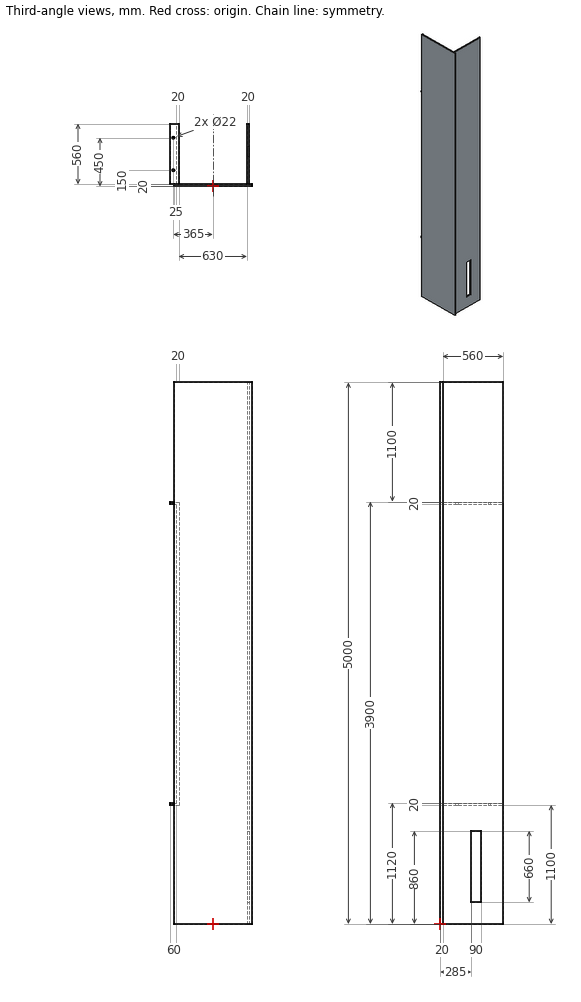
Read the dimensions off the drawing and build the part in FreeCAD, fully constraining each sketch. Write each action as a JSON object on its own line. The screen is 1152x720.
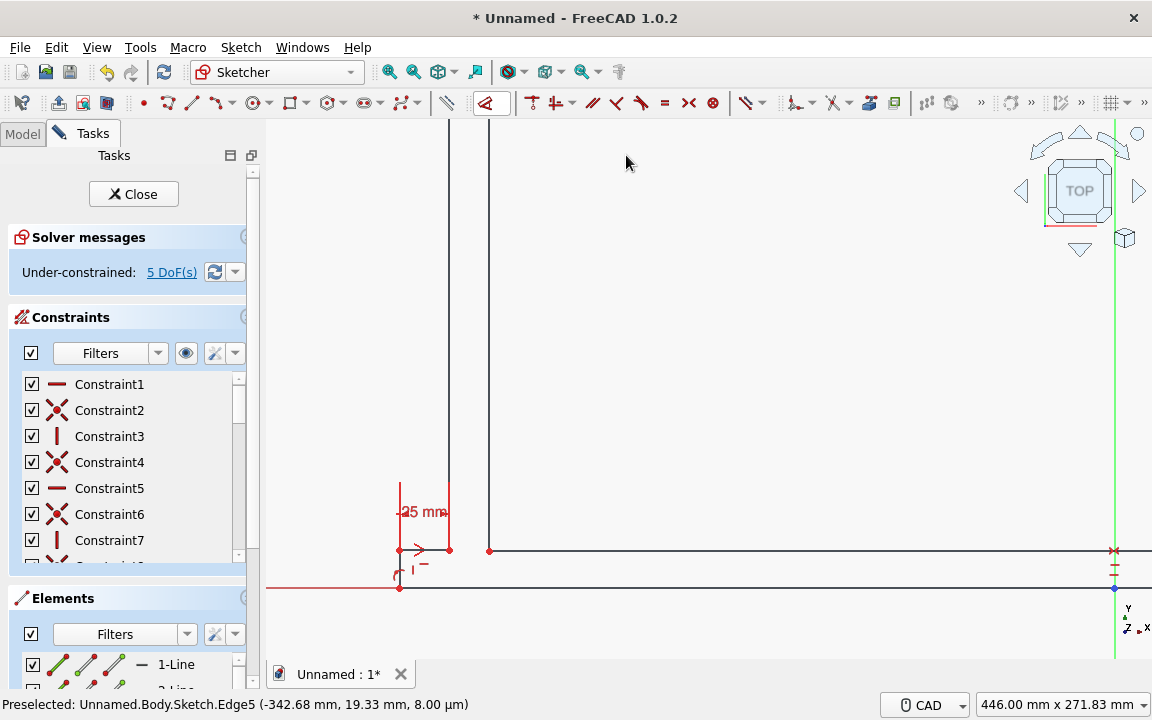
{"action": "left_click", "coordinate": [400, 562]}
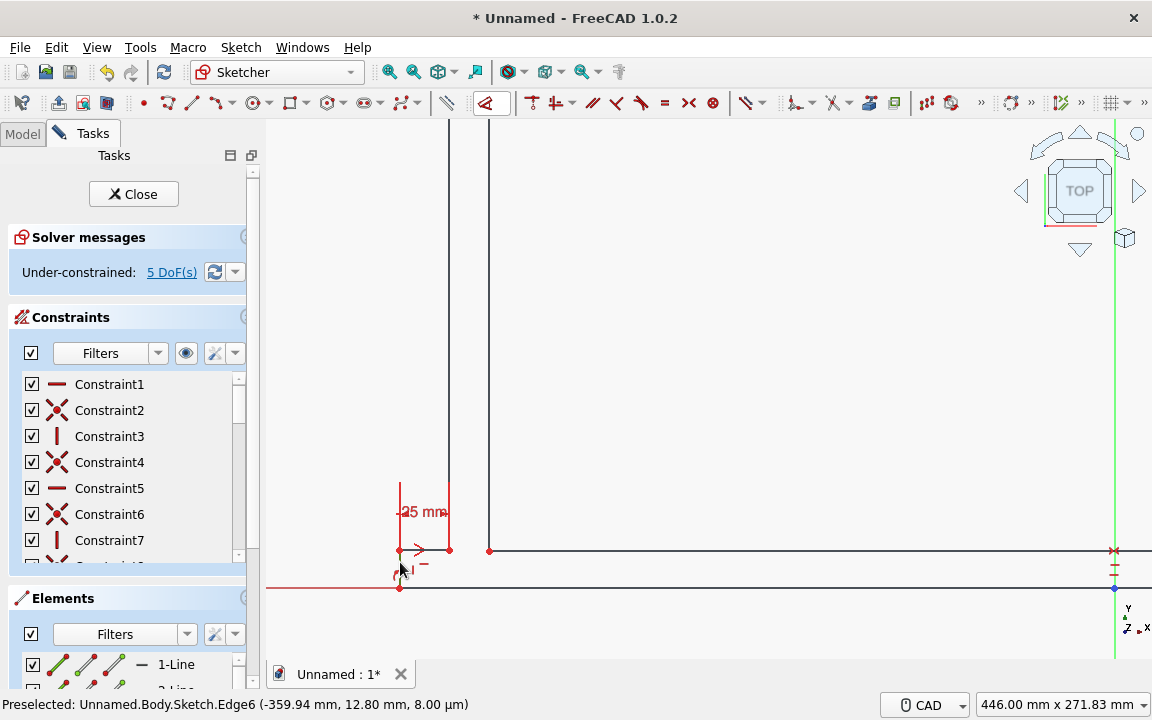
{"action": "left_click", "coordinate": [504, 104]}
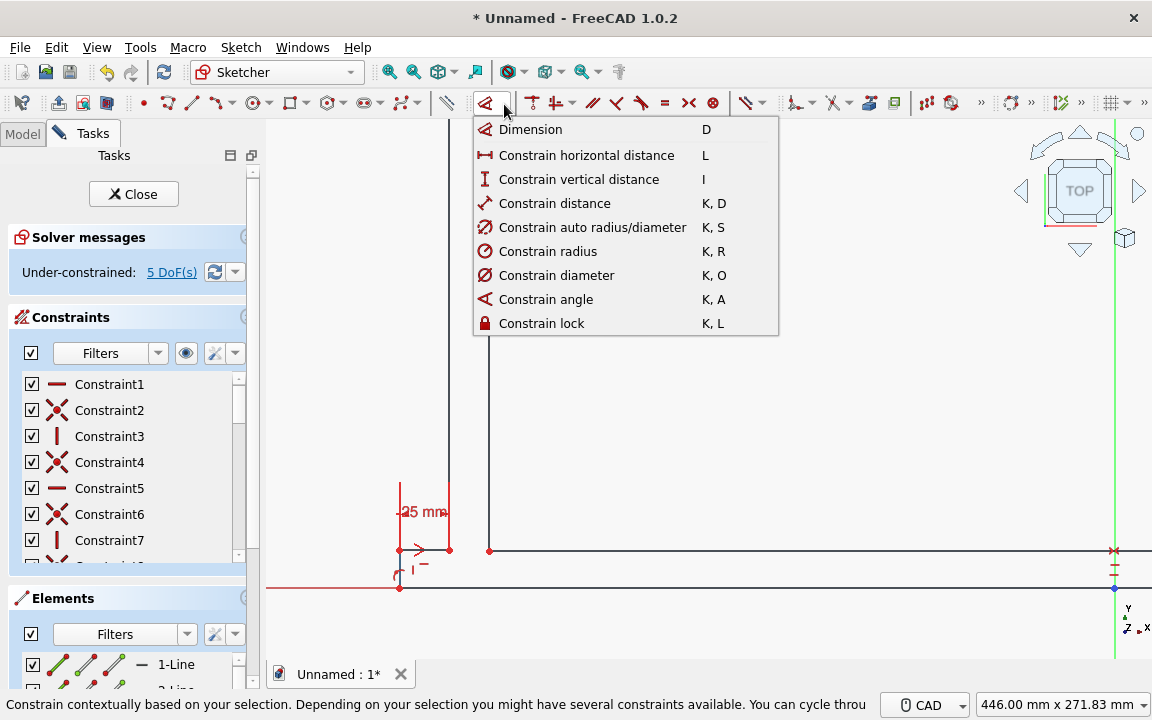
{"action": "left_click", "coordinate": [626, 179]}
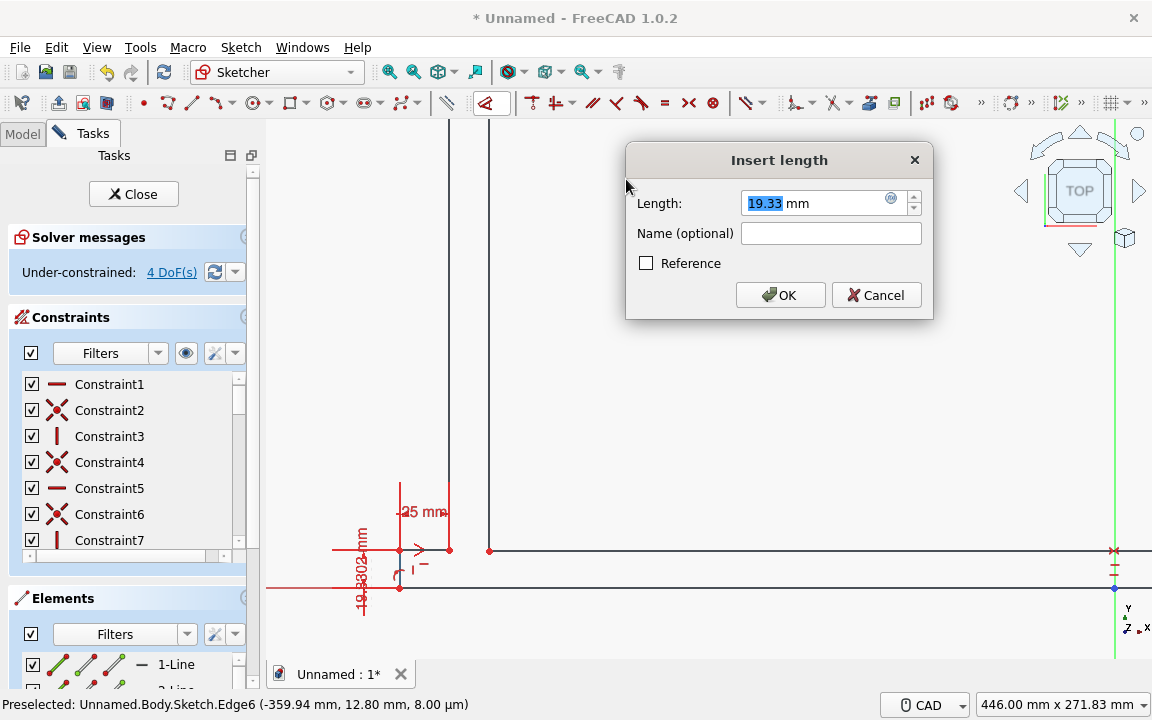
{"action": "type", "text": "20"}
{"action": "key", "text": "Return"}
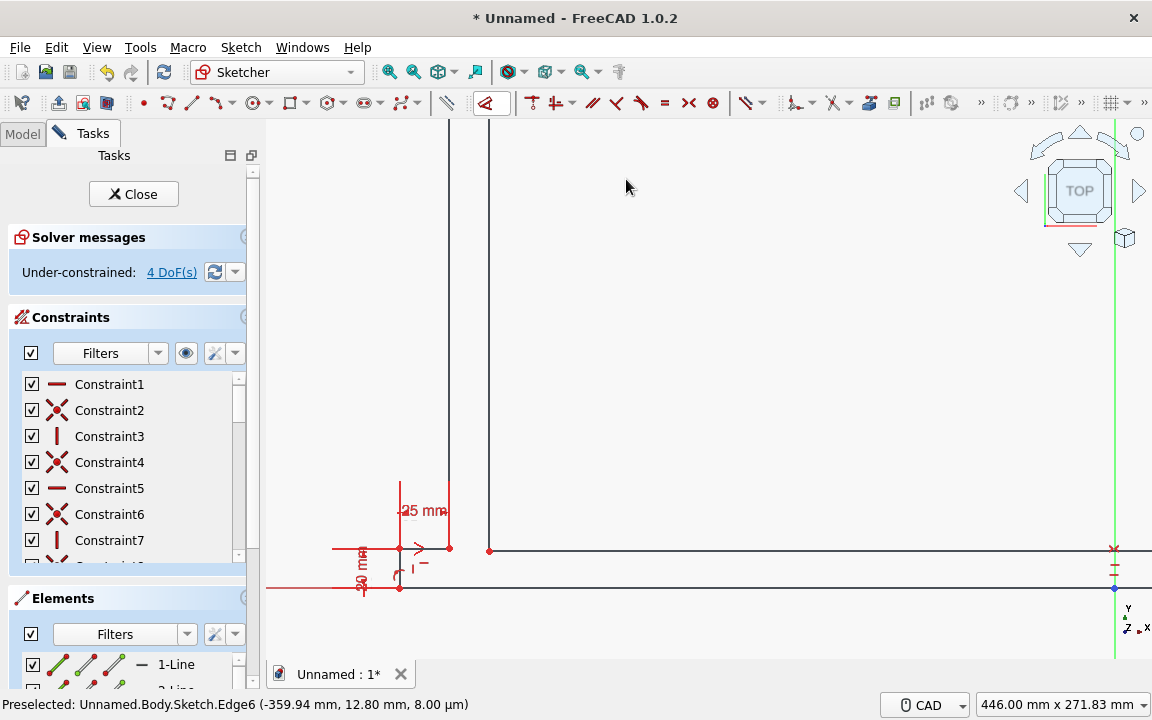
{"action": "scroll", "coordinate": [436, 551], "scroll_direction": "down", "scroll_amount": 6}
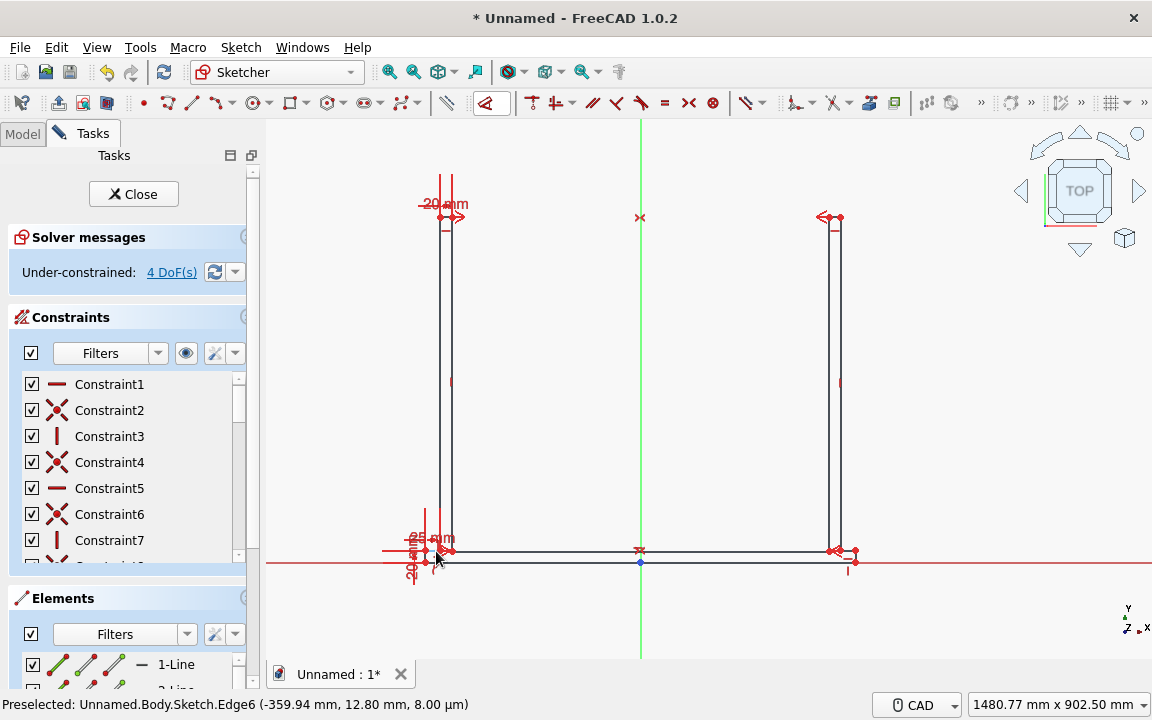
{"action": "scroll", "coordinate": [837, 217], "scroll_direction": "up", "scroll_amount": 7}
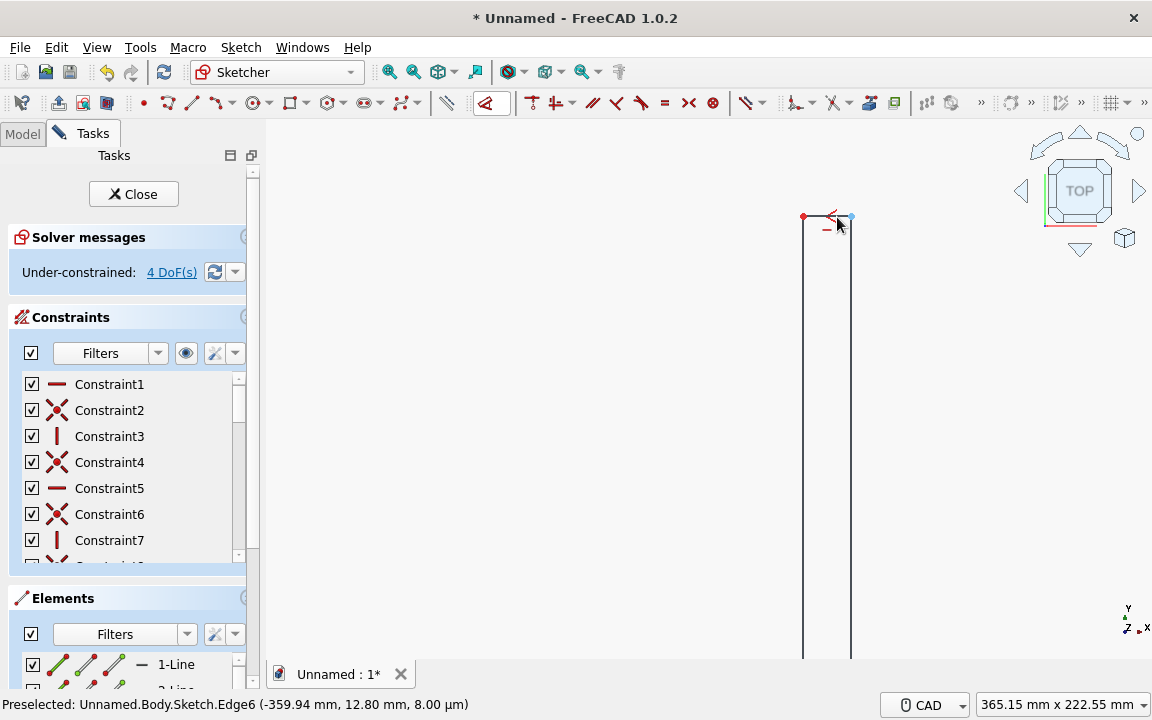
{"action": "left_click", "coordinate": [837, 216]}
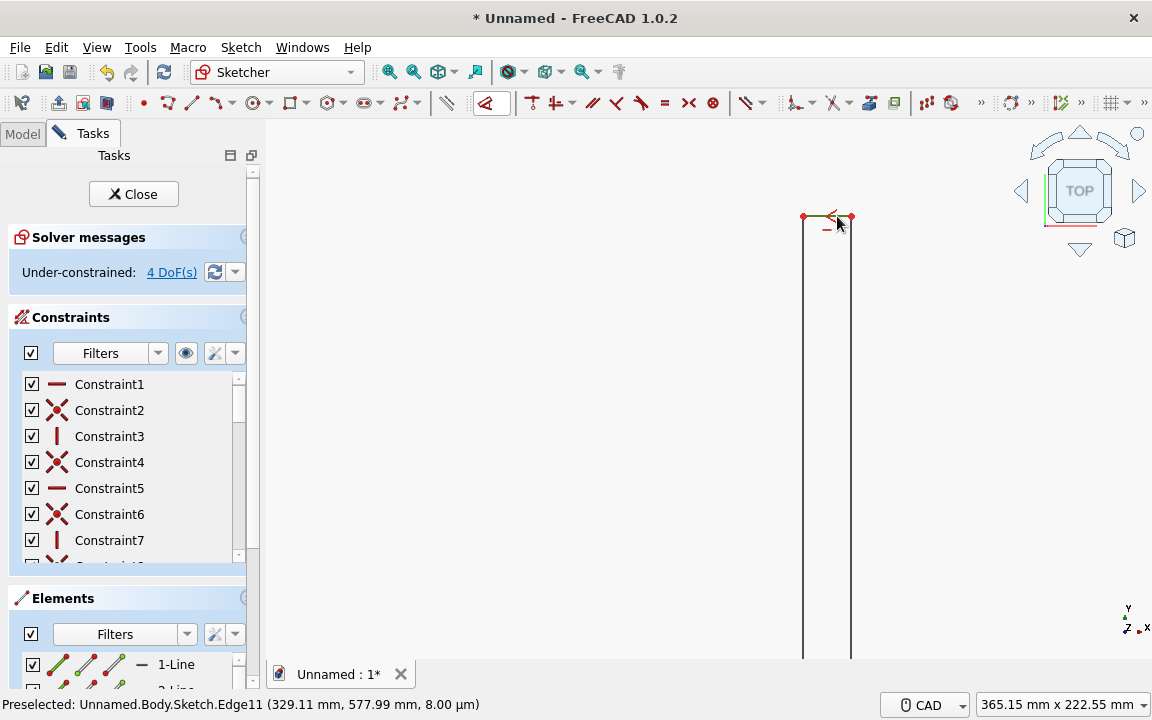
{"action": "left_click", "coordinate": [504, 104]}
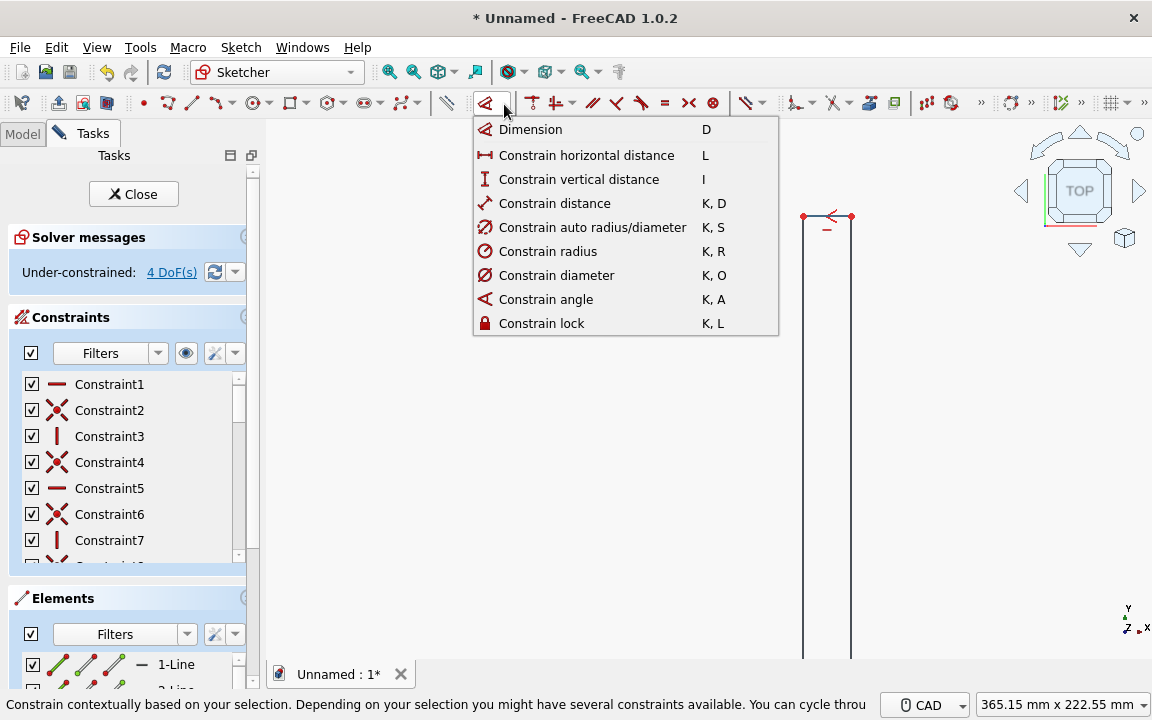
{"action": "left_click", "coordinate": [626, 155]}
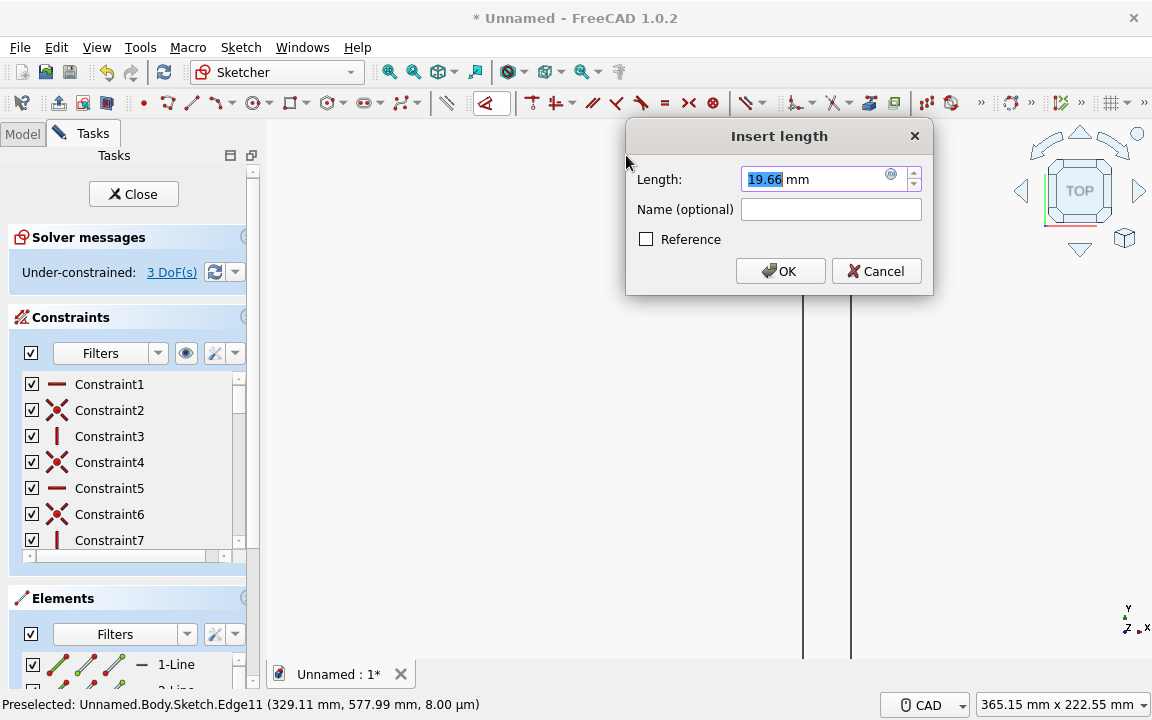
{"action": "type", "text": "20"}
{"action": "key", "text": "Return"}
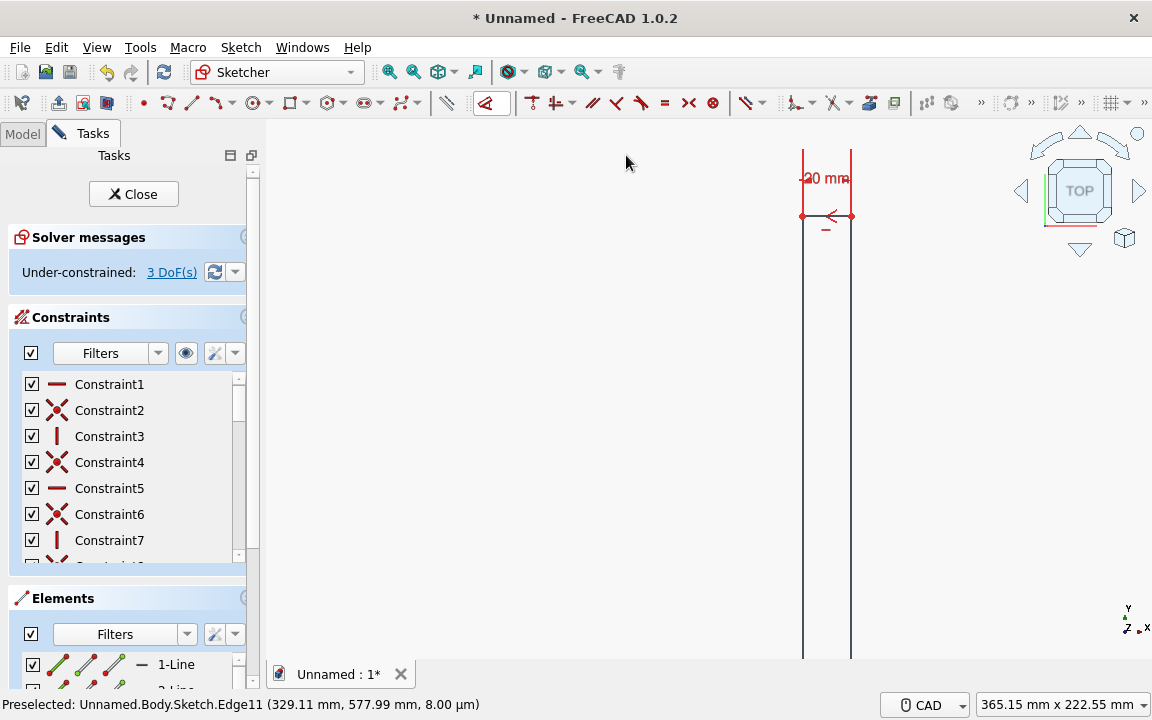
{"action": "scroll", "coordinate": [838, 217], "scroll_direction": "down", "scroll_amount": 7}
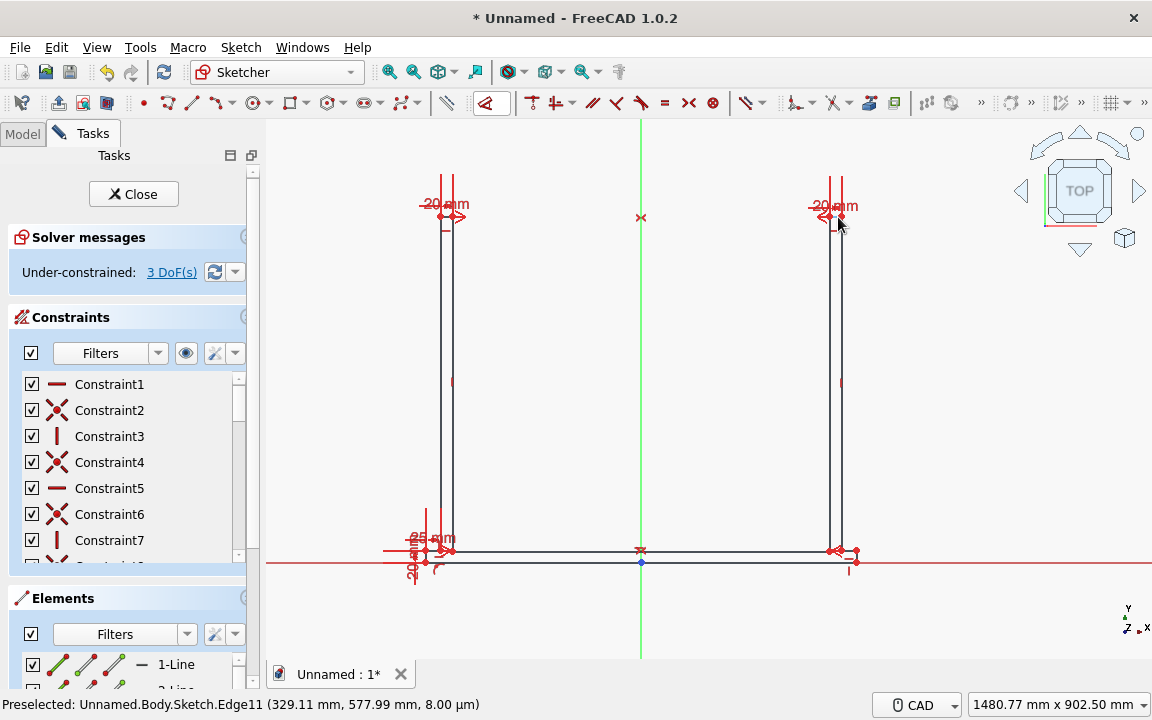
{"action": "scroll", "coordinate": [717, 552], "scroll_direction": "up", "scroll_amount": 2}